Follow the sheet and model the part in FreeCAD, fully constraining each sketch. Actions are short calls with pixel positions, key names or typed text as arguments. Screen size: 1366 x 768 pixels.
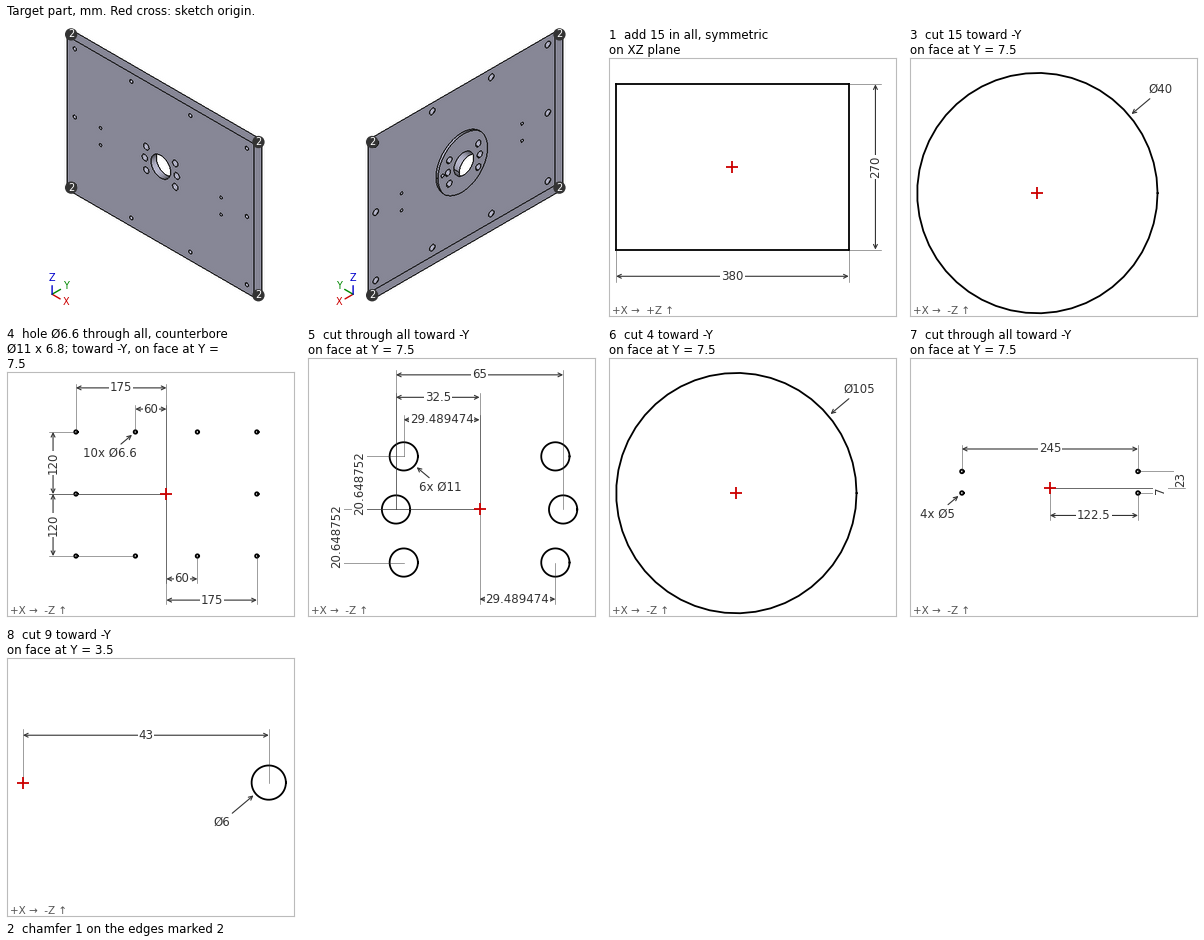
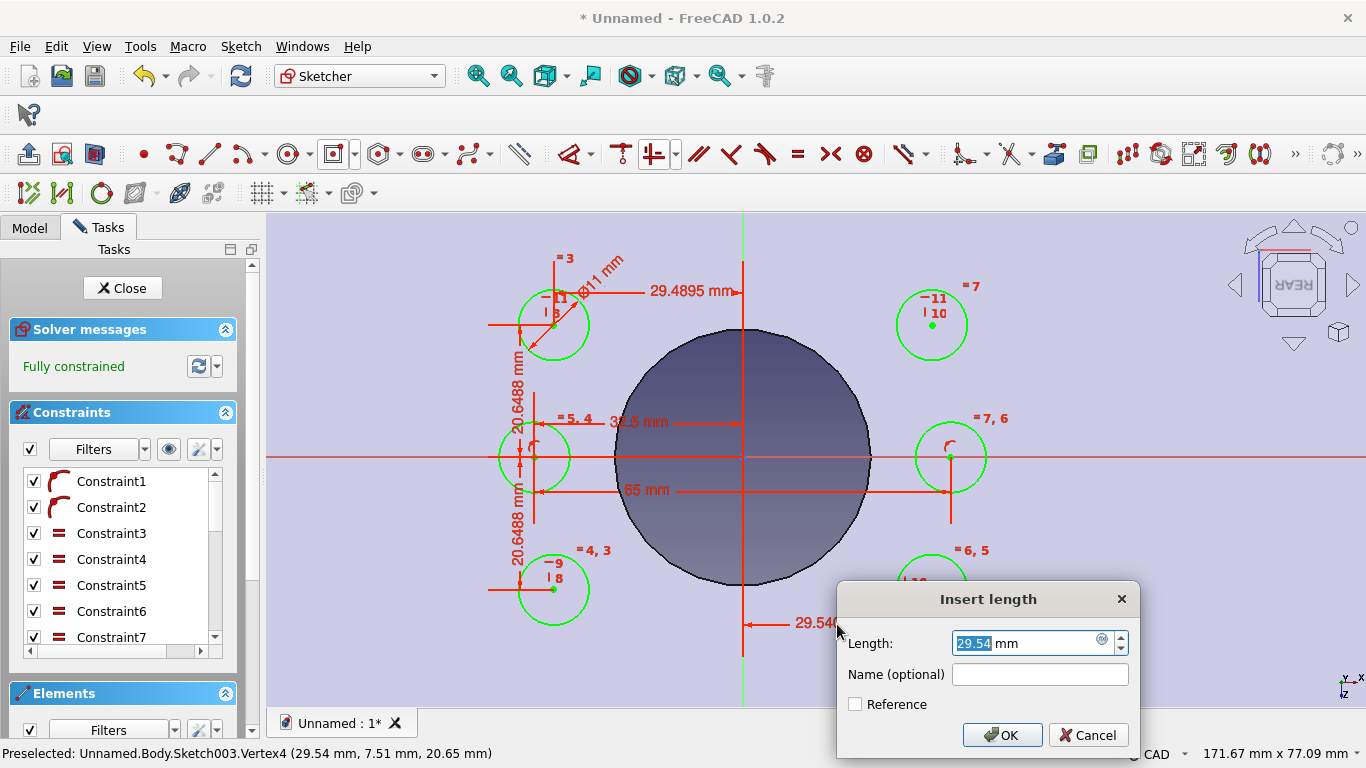
text(29.489474)
key(Return)
key(Escape)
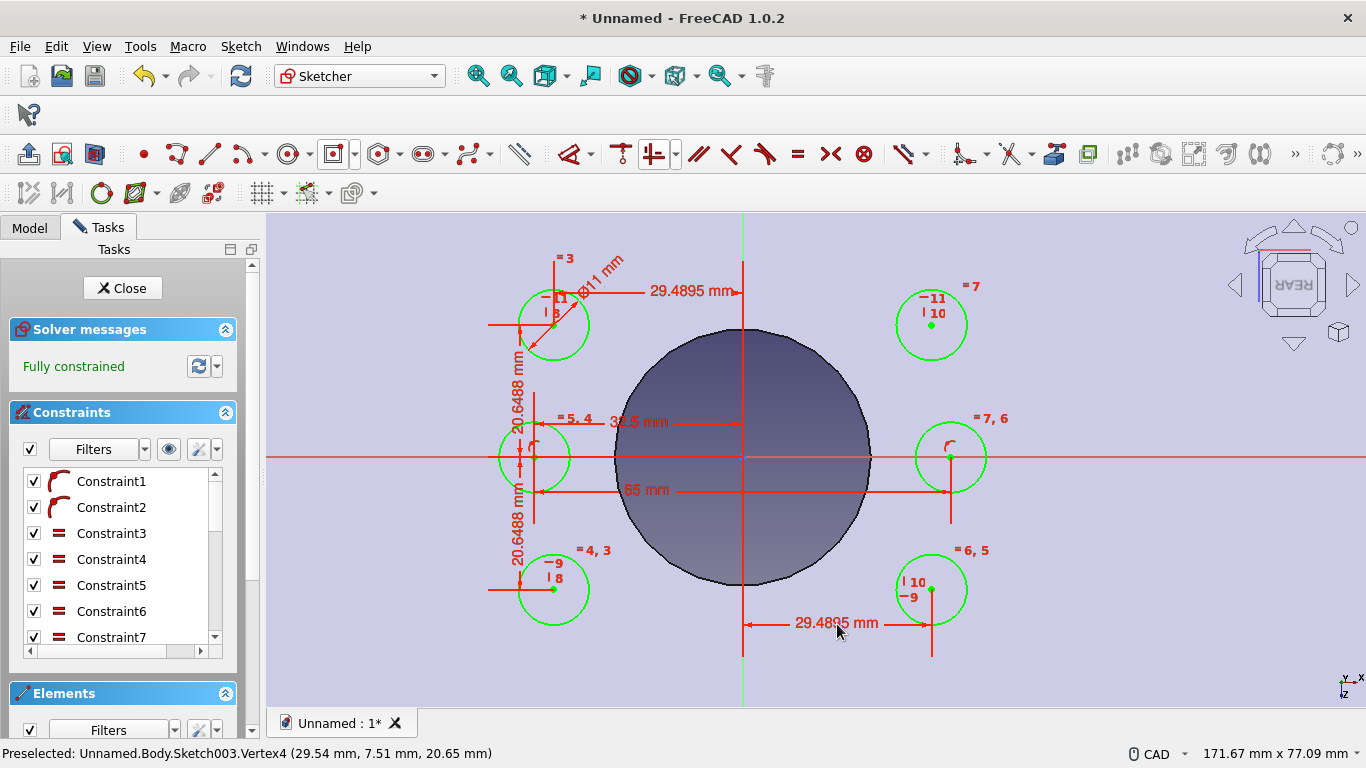
click(123, 288)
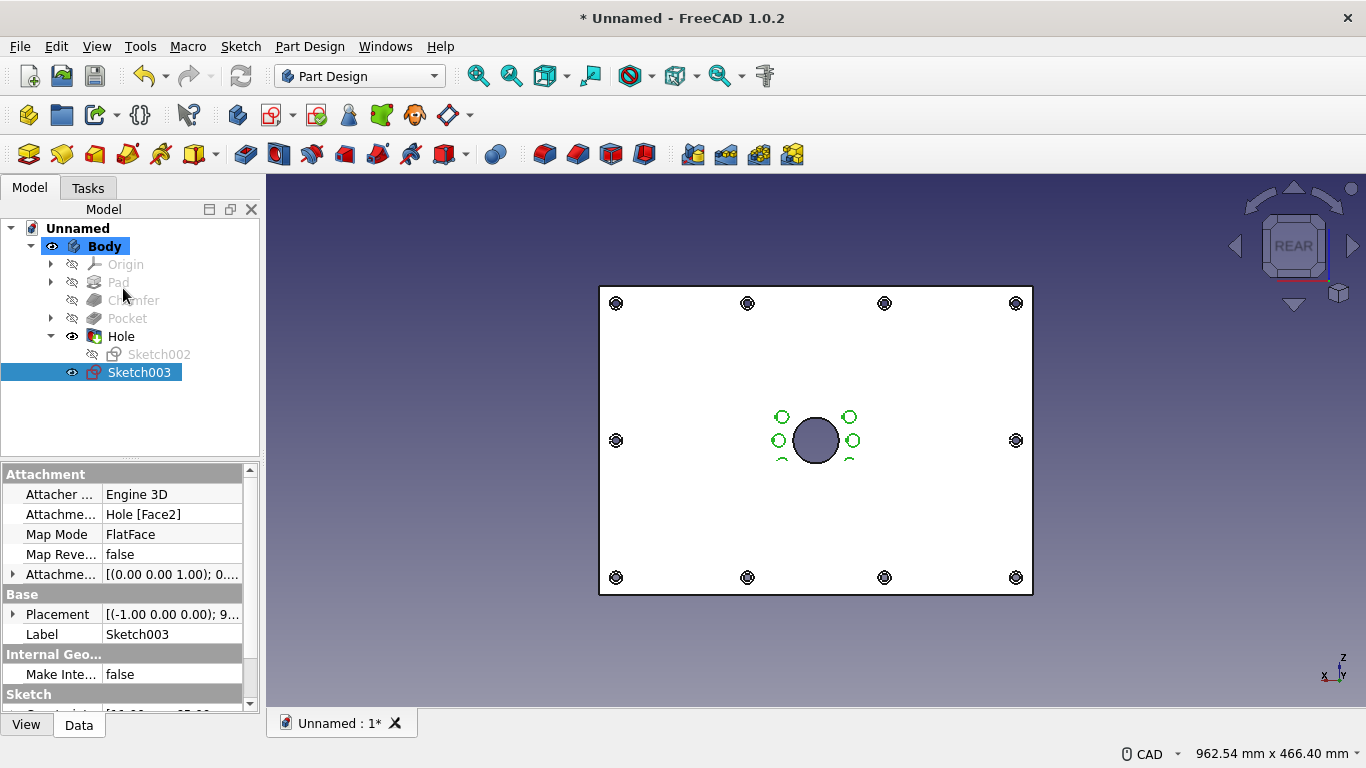
click(246, 154)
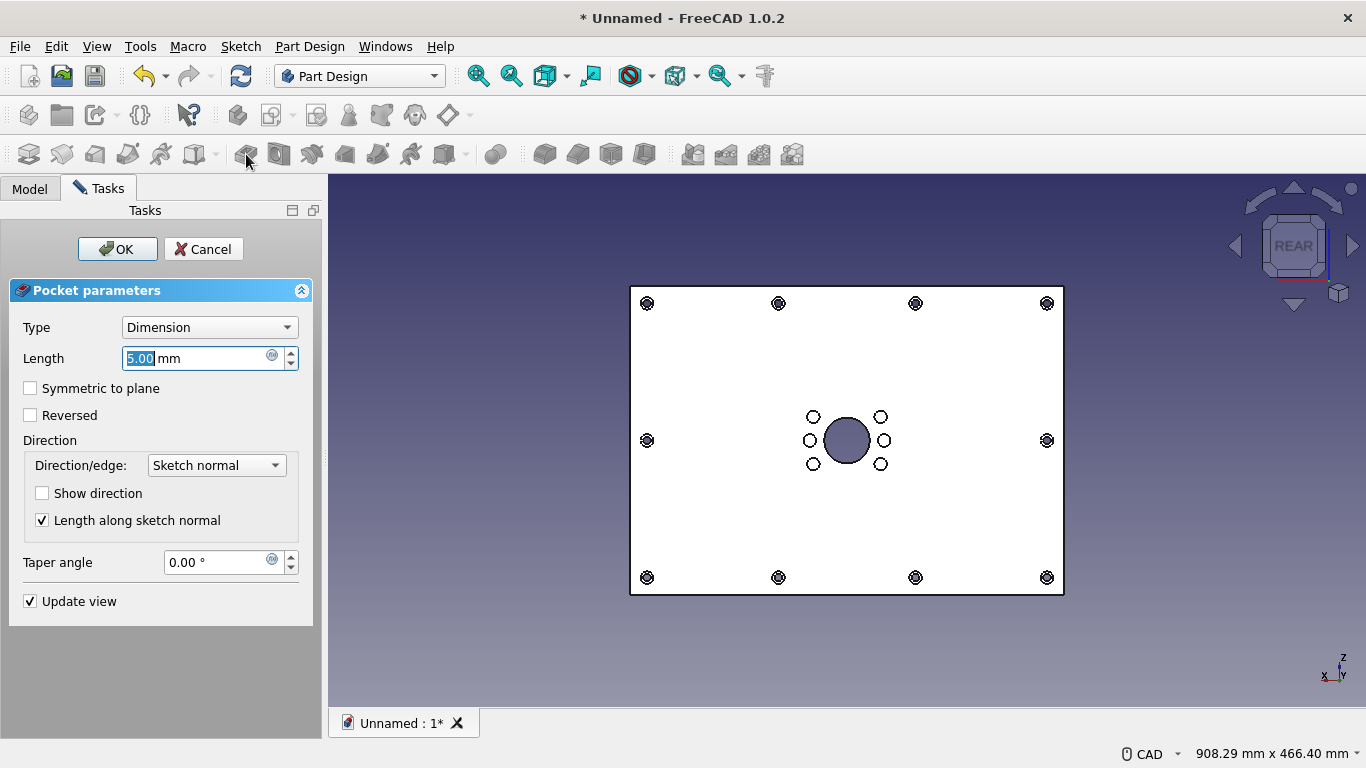
click(210, 328)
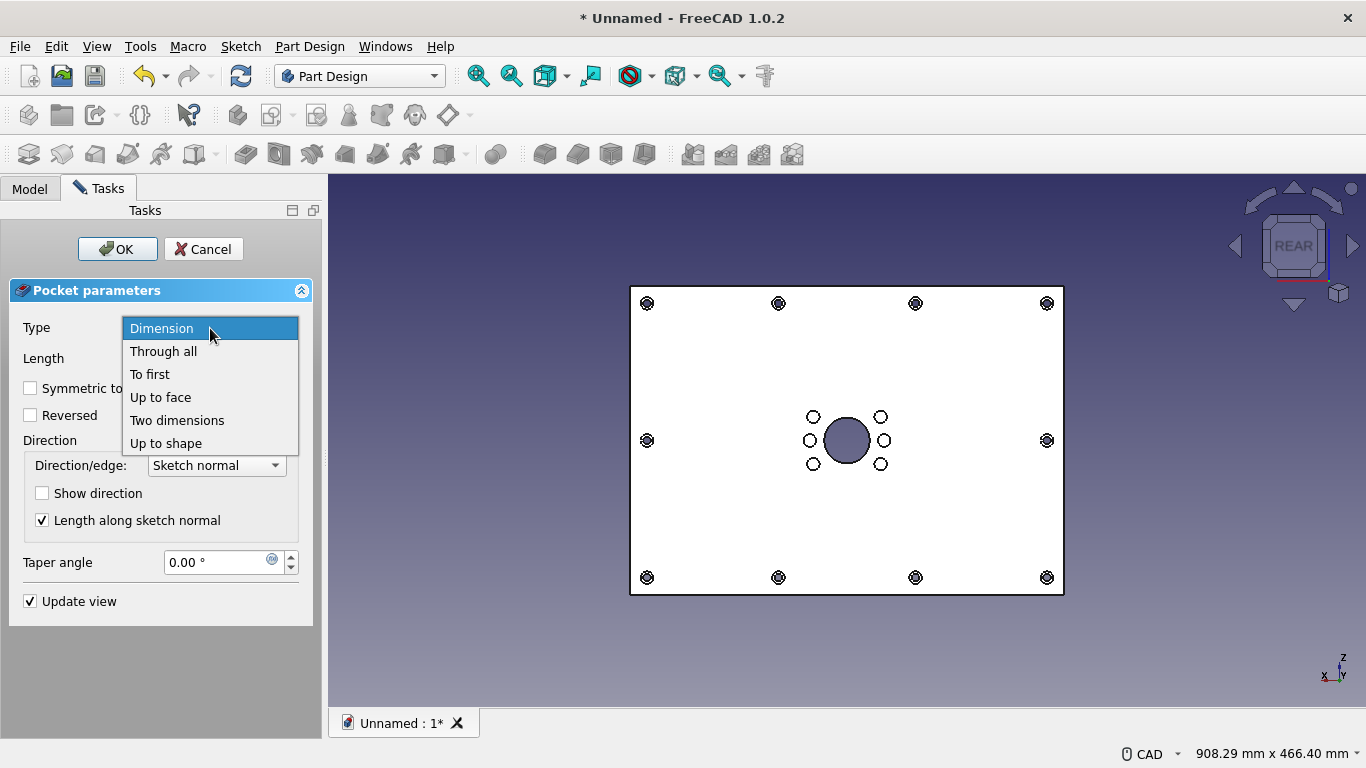
click(208, 352)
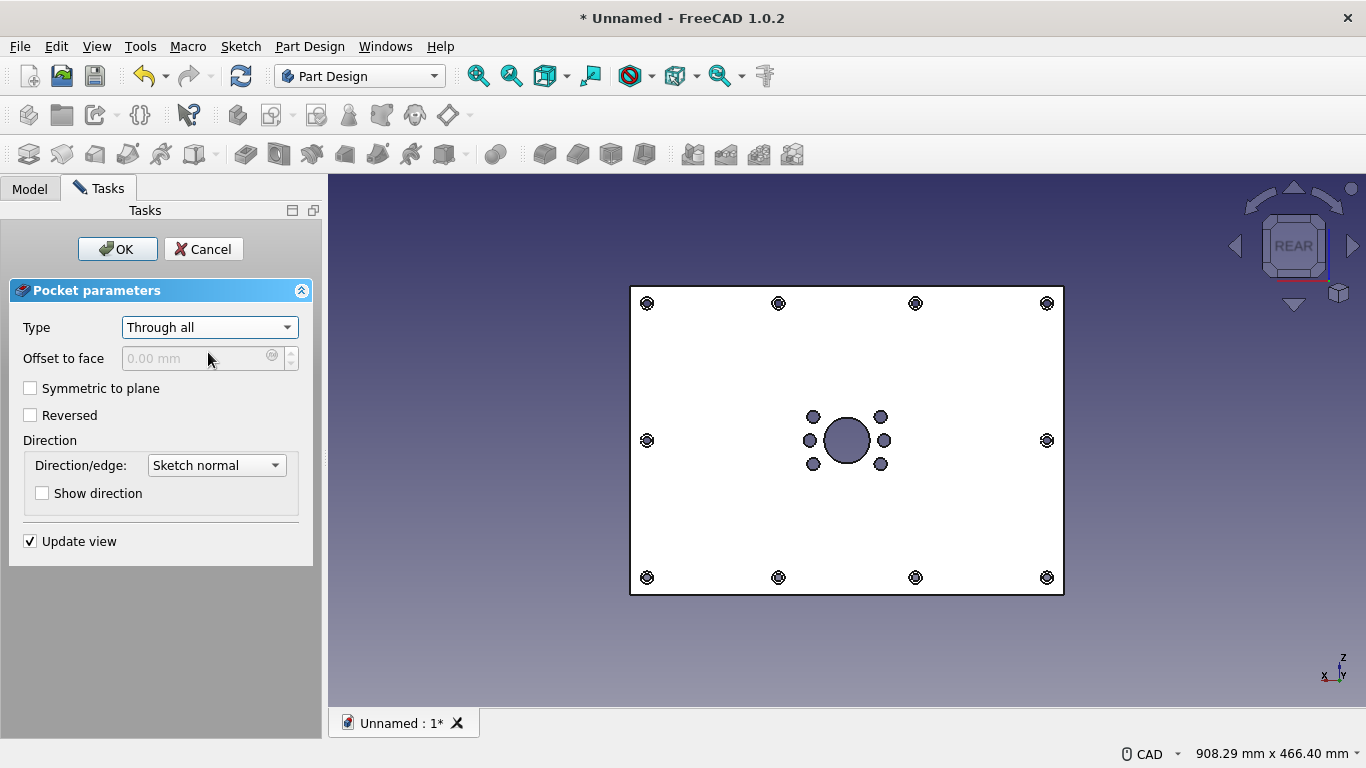
click(118, 249)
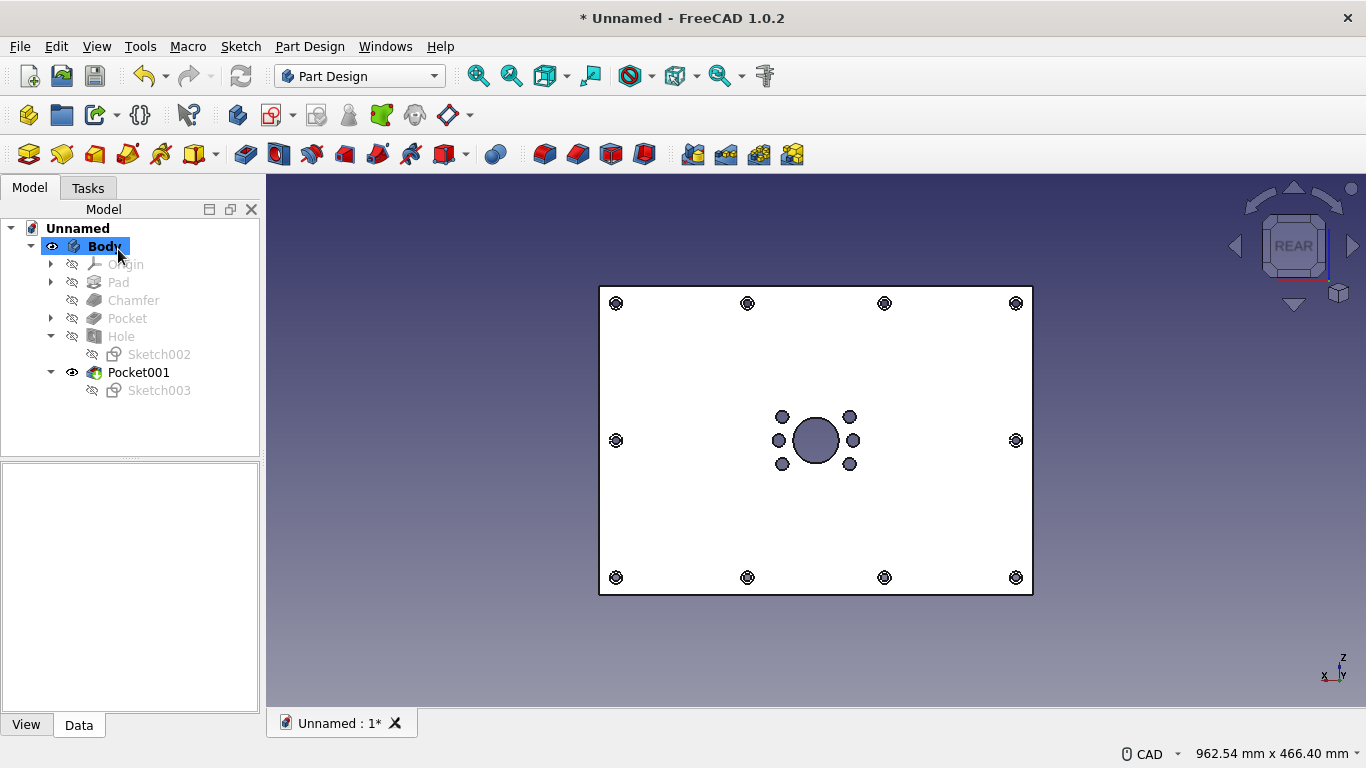
click(692, 395)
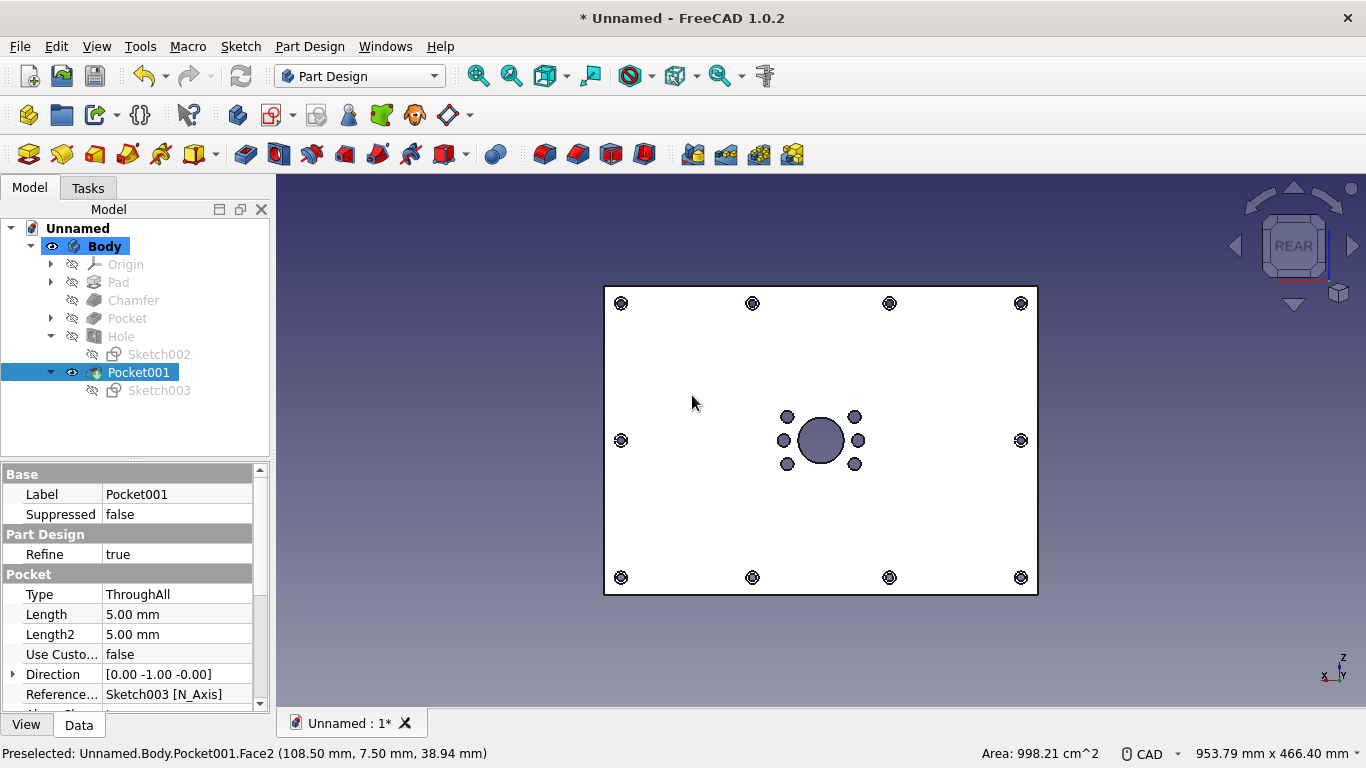
click(270, 116)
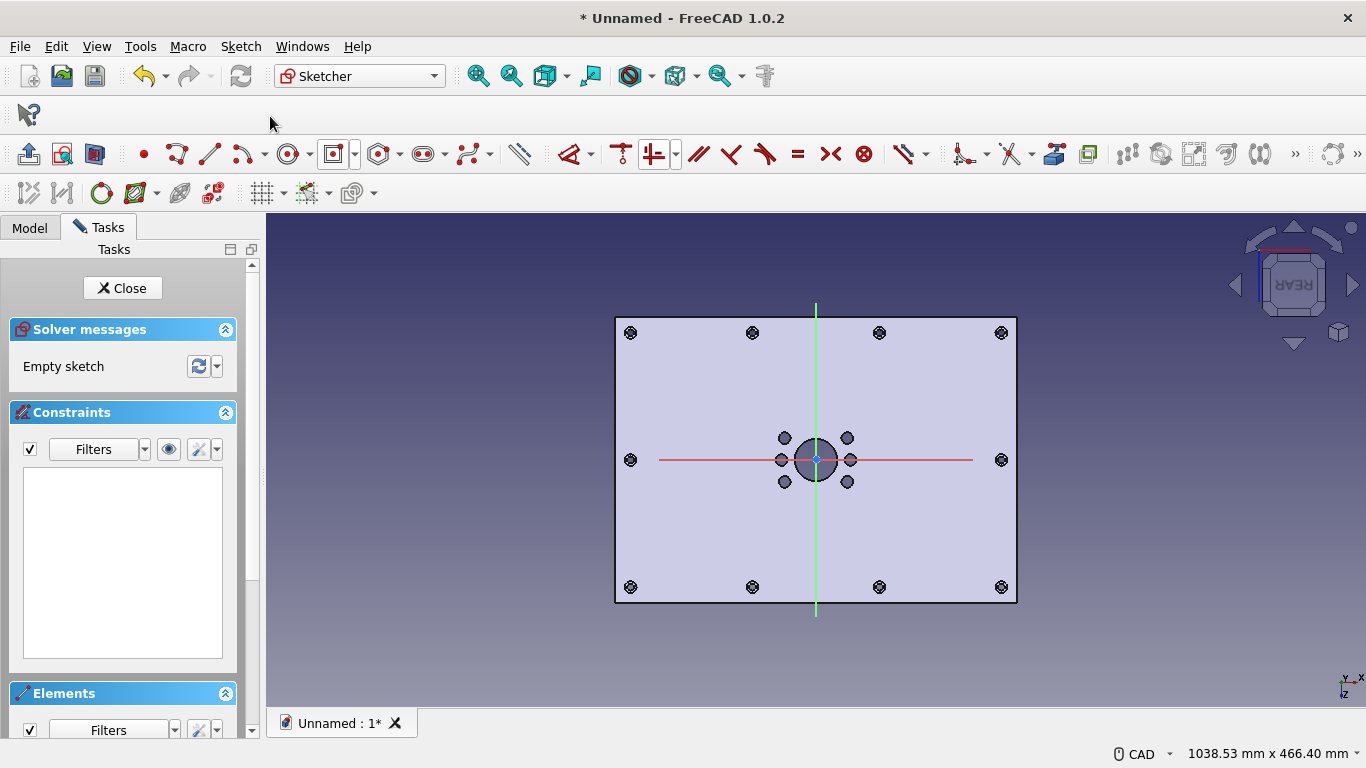
scroll(856, 460, up, 5)